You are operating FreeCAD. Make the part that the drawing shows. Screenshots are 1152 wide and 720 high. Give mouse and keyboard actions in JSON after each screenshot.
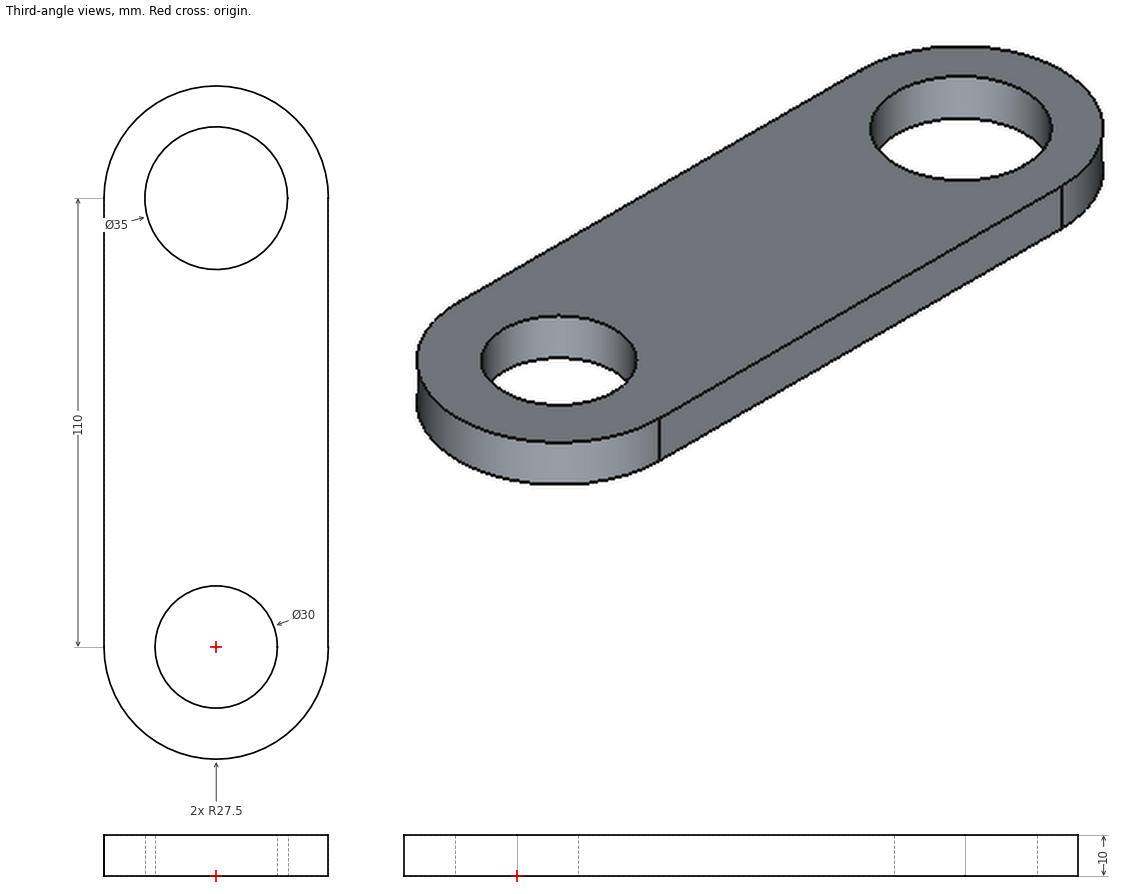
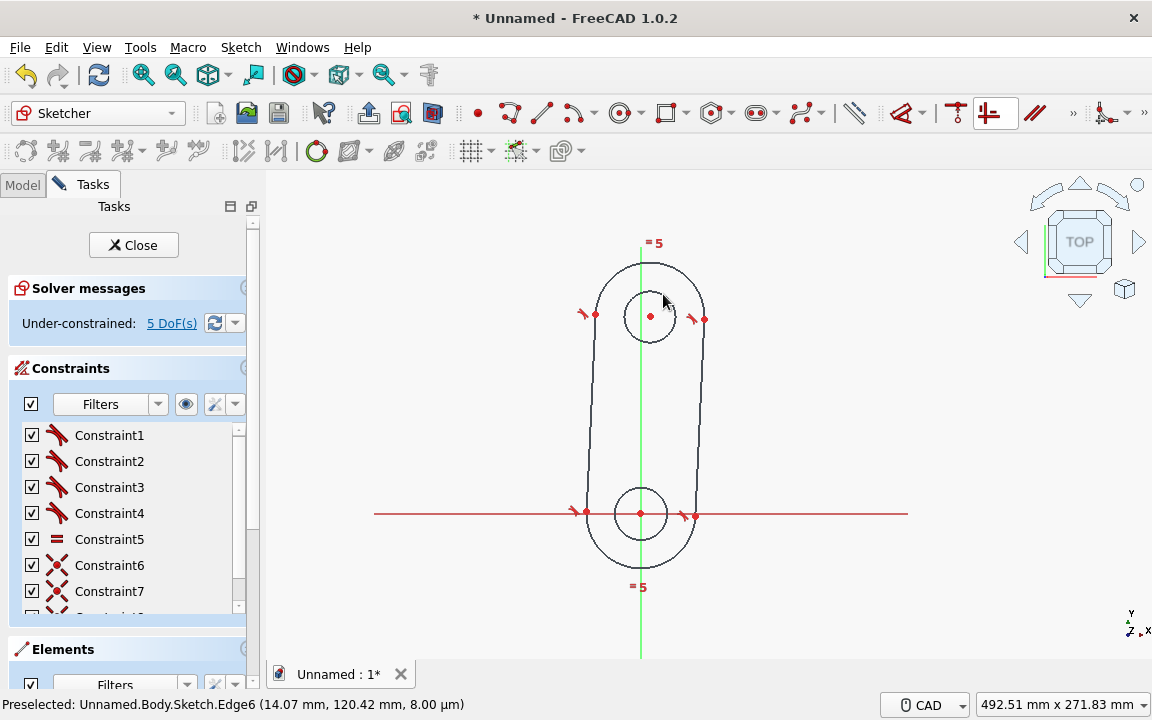
{"action": "left_click", "coordinate": [589, 452]}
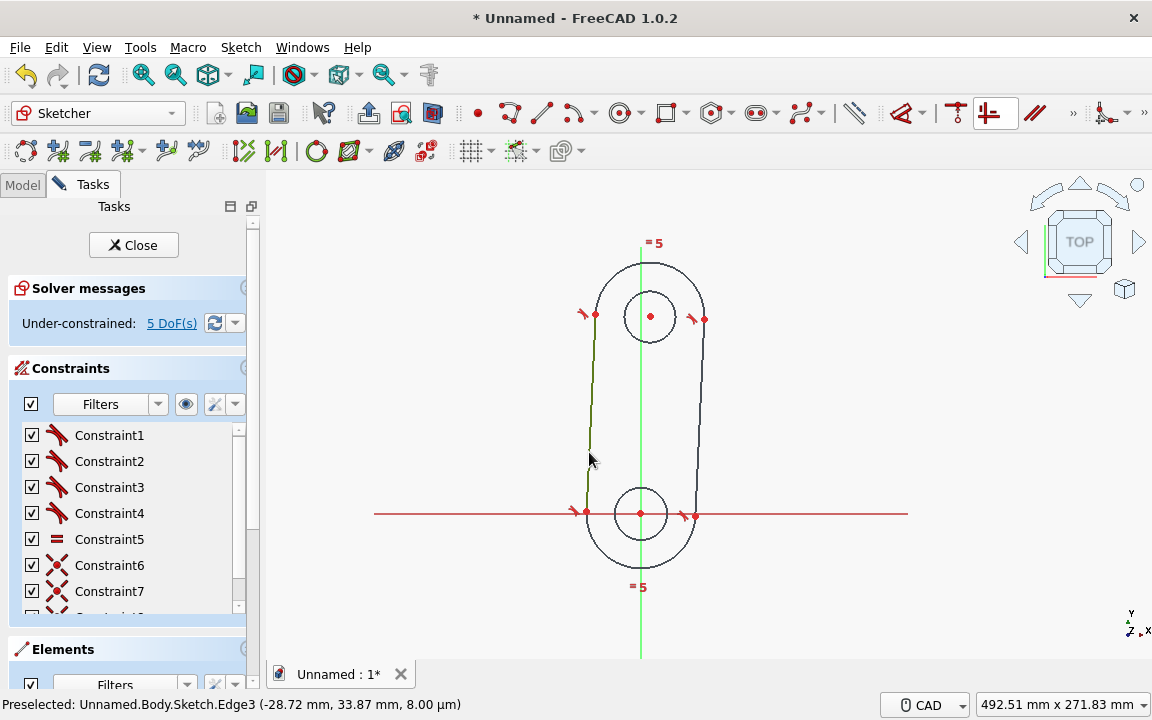
{"action": "key", "text": "v"}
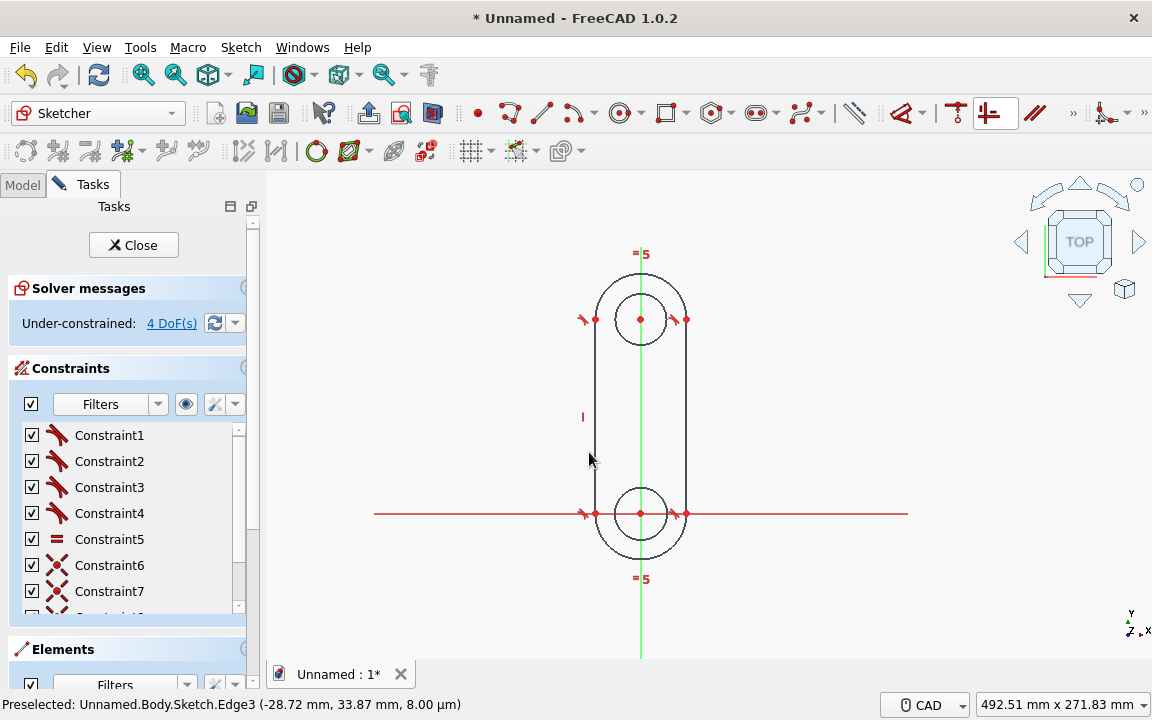
{"action": "left_click", "coordinate": [902, 114]}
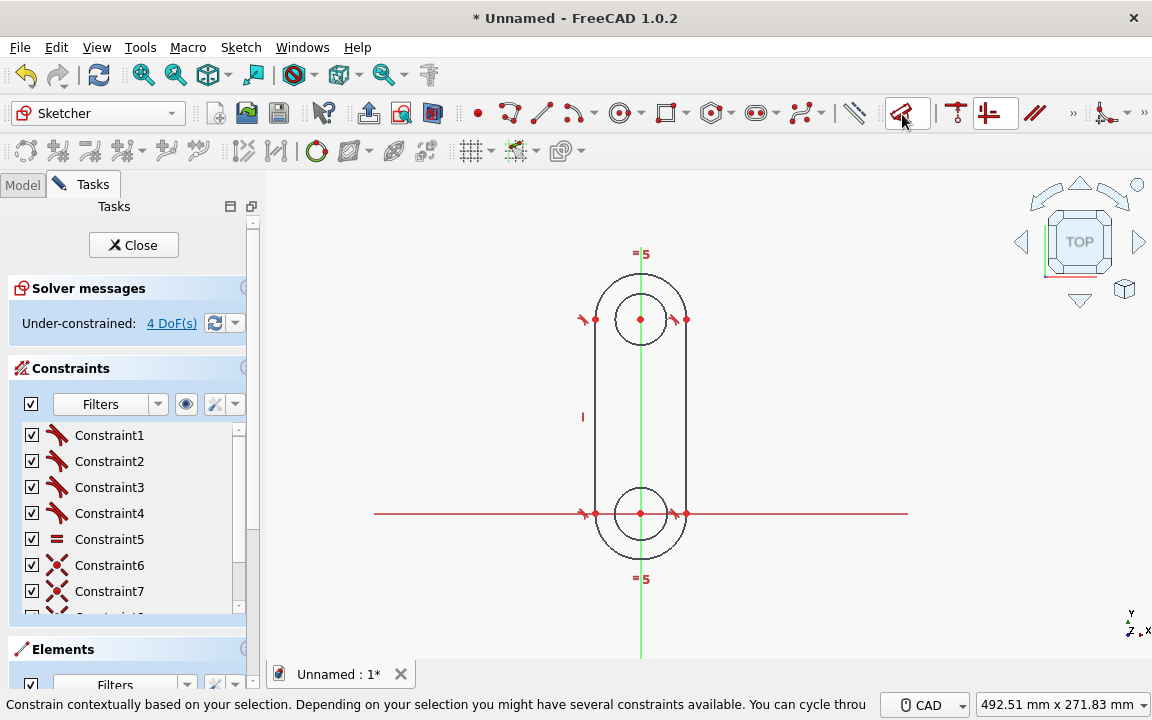
{"action": "left_click", "coordinate": [614, 551]}
{"action": "left_click", "coordinate": [595, 577]}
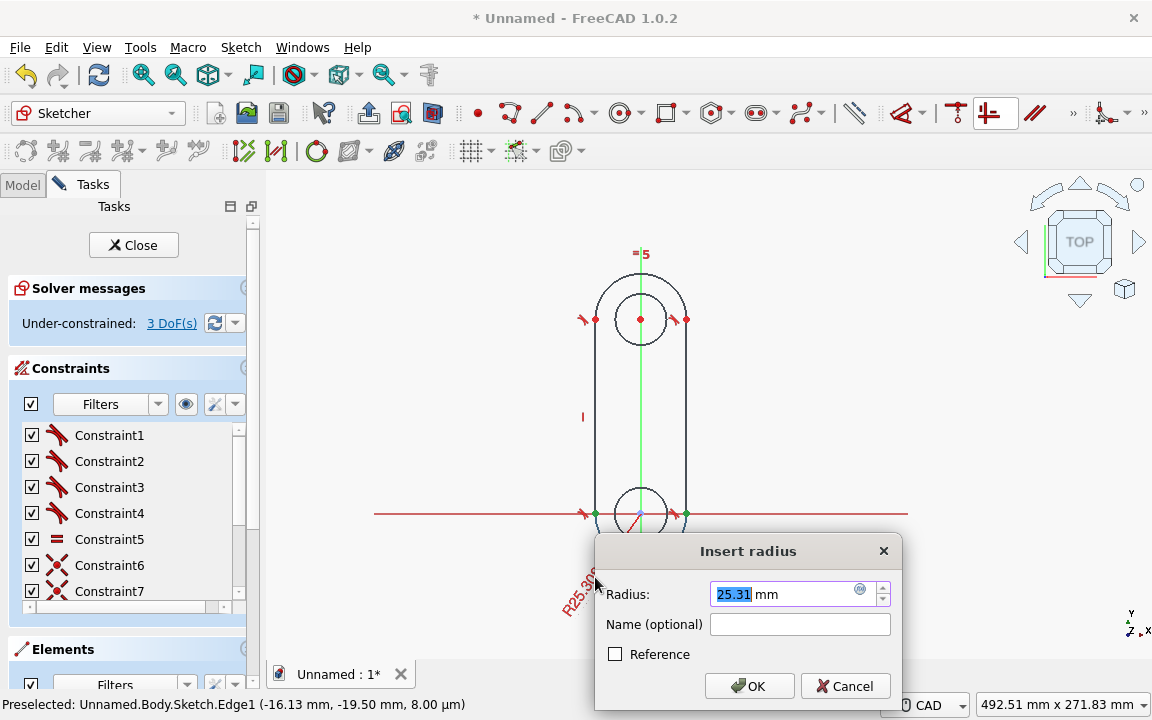
{"action": "type", "text": "27.5"}
{"action": "key", "text": "Return"}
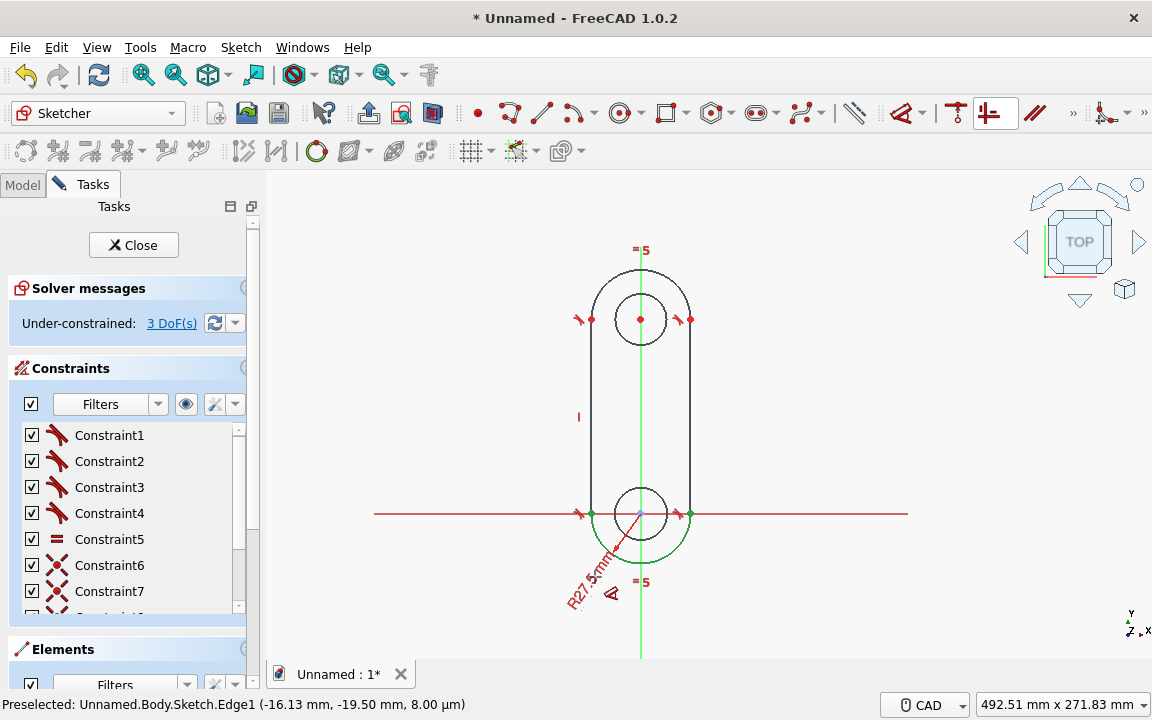
{"action": "left_click", "coordinate": [659, 495]}
{"action": "left_click", "coordinate": [656, 458]}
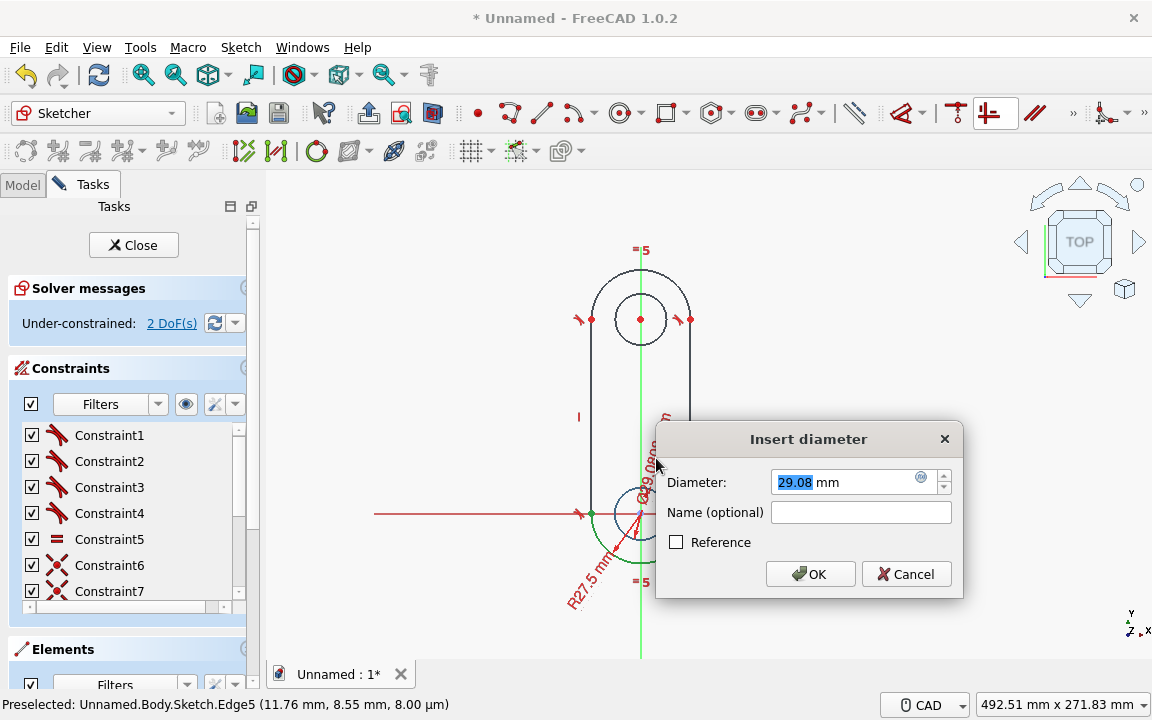
{"action": "type", "text": "30"}
{"action": "key", "text": "Return"}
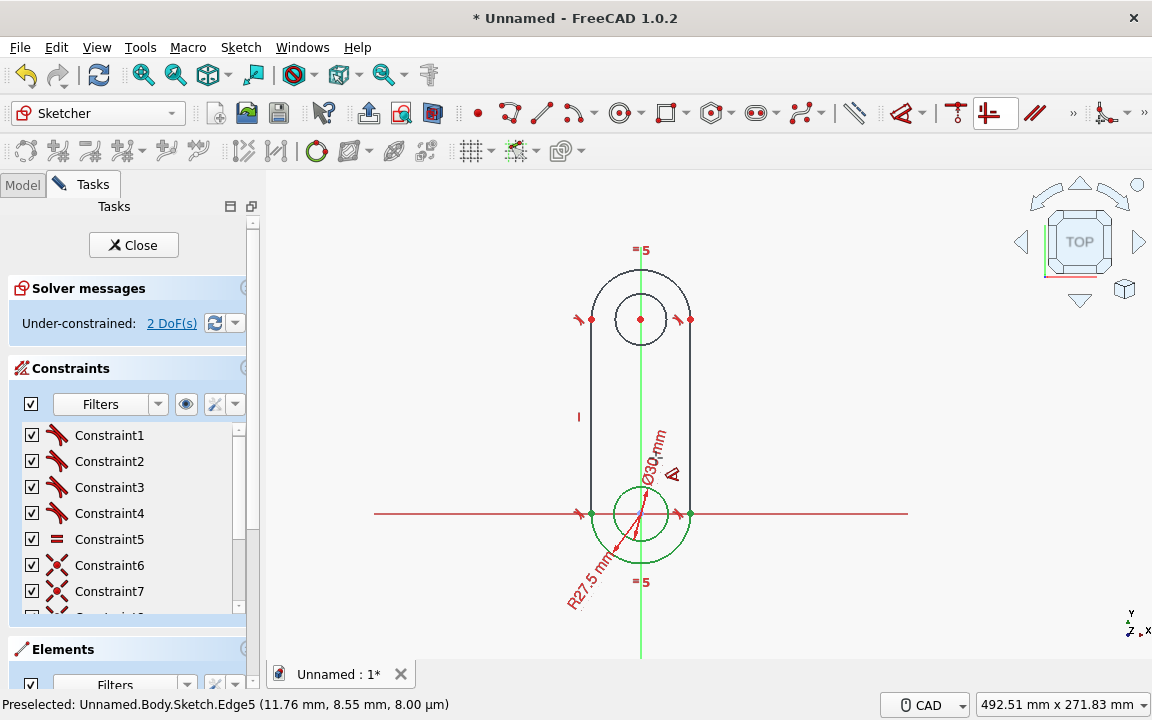
{"action": "left_click", "coordinate": [659, 301]}
{"action": "left_click", "coordinate": [697, 262]}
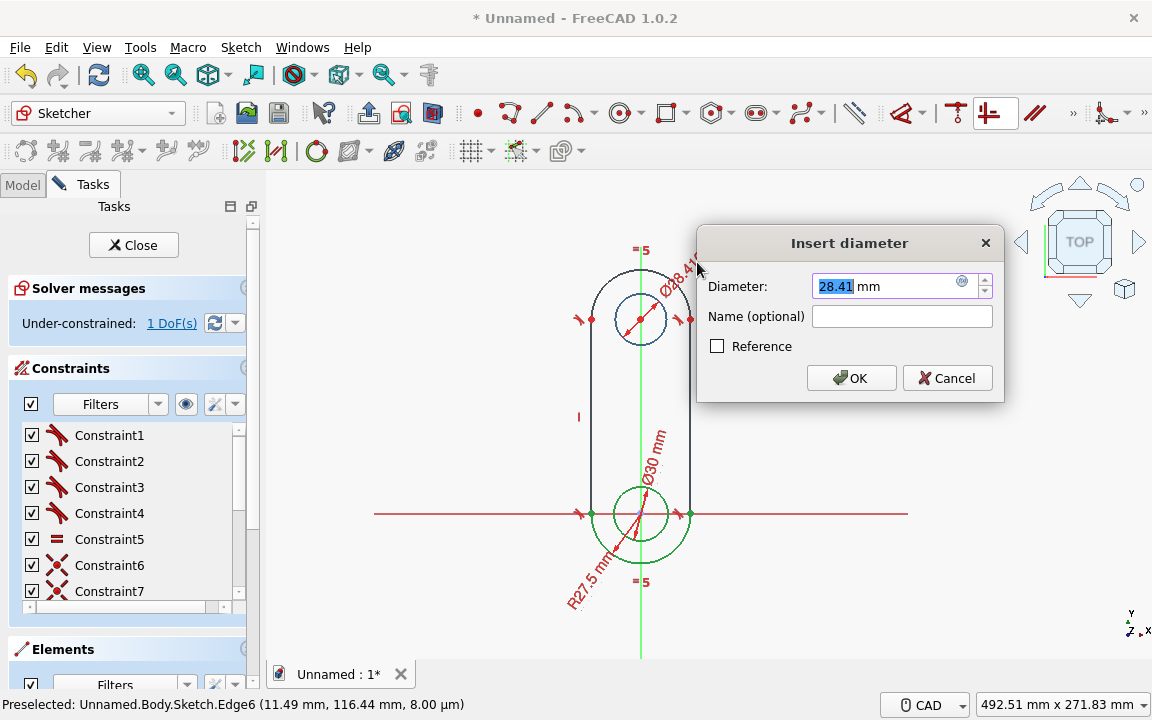
{"action": "type", "text": "35"}
{"action": "key", "text": "Return"}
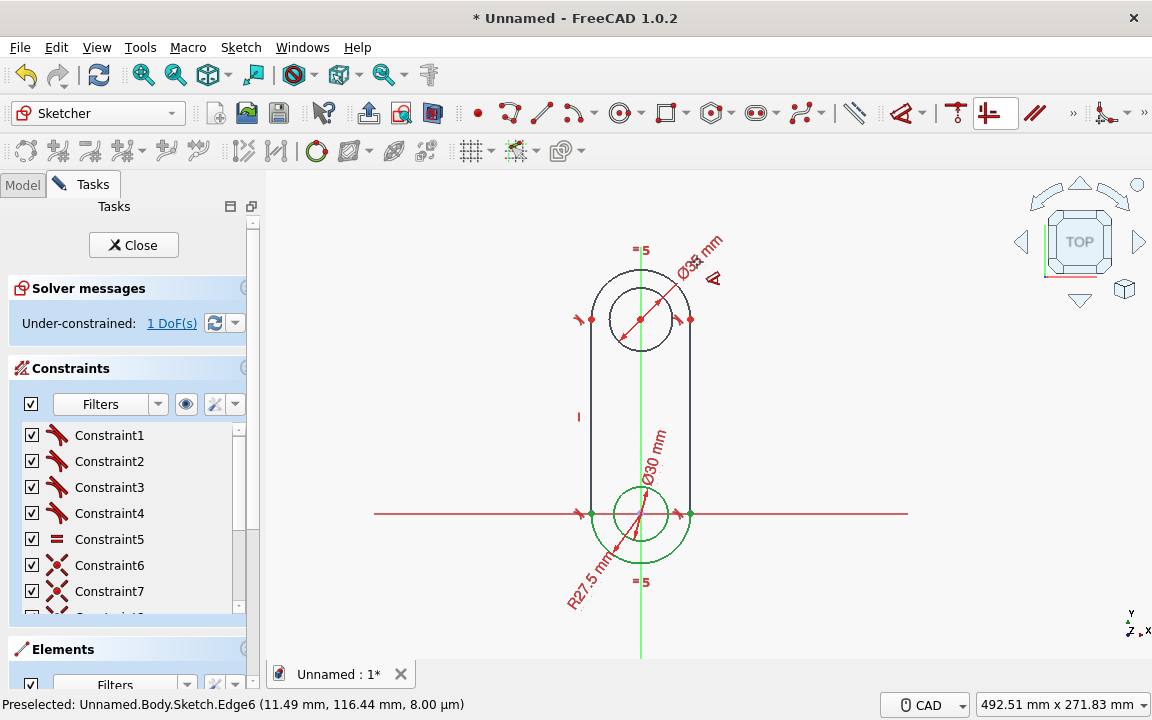
{"action": "left_click", "coordinate": [591, 456]}
{"action": "left_click", "coordinate": [557, 417]}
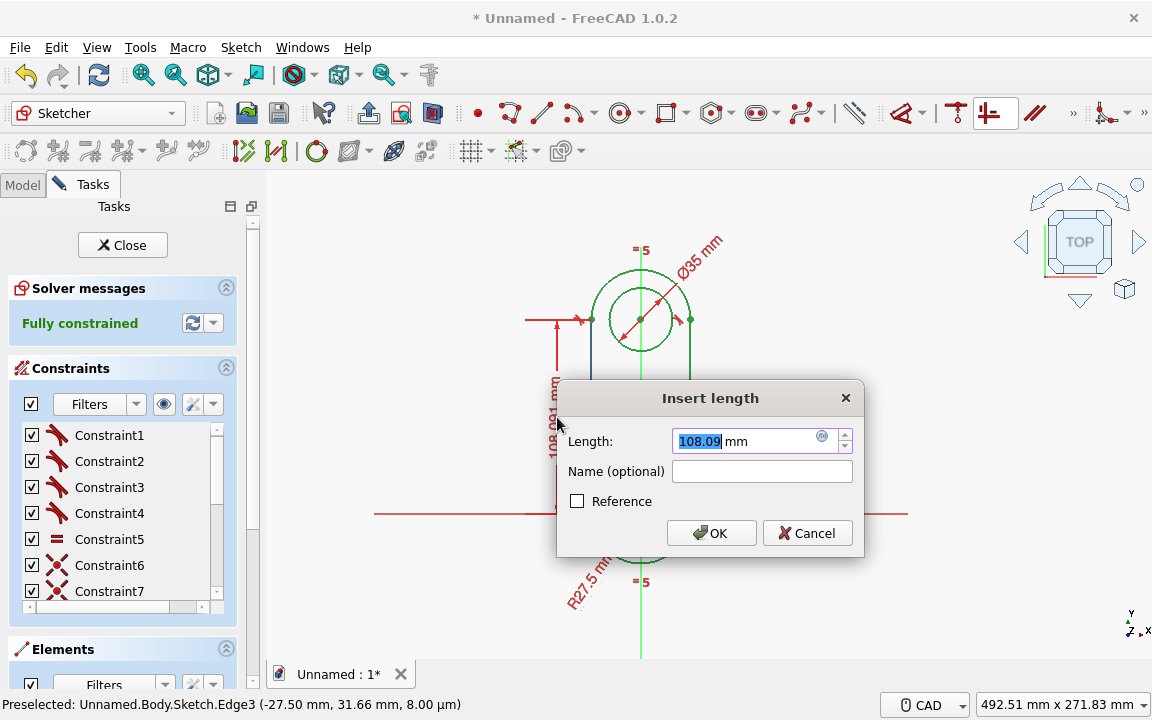
{"action": "type", "text": "110"}
{"action": "key", "text": "Return"}
{"action": "key", "text": "Escape"}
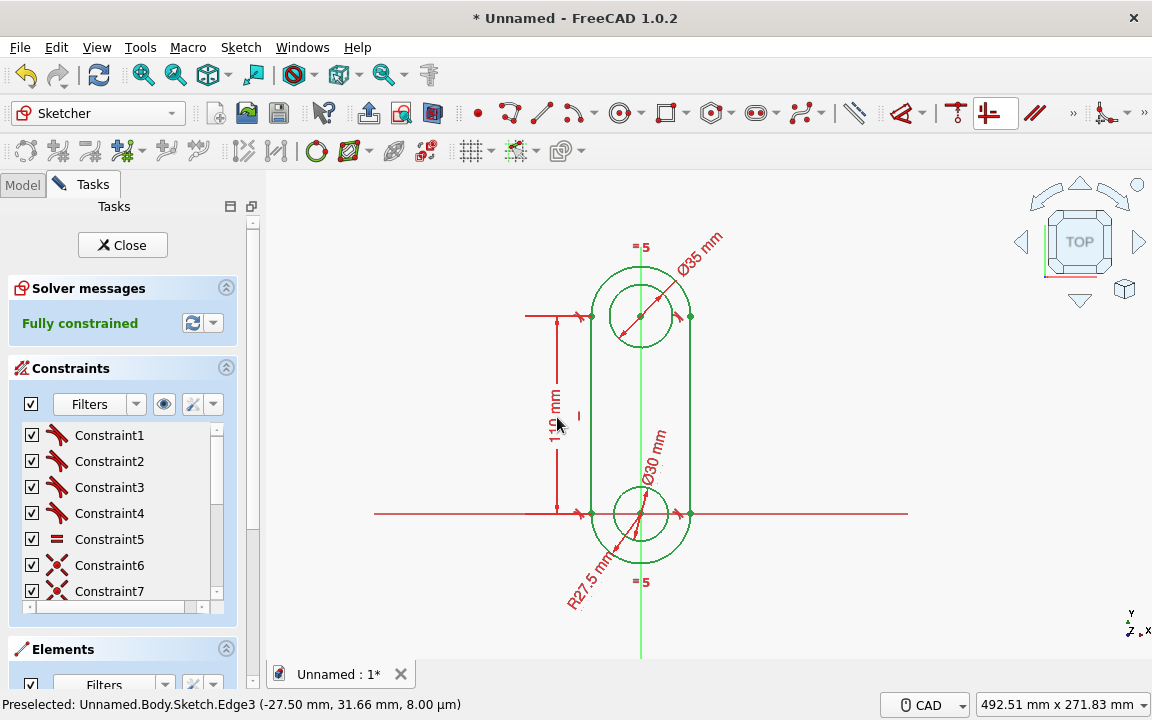
{"action": "left_click", "coordinate": [123, 245]}